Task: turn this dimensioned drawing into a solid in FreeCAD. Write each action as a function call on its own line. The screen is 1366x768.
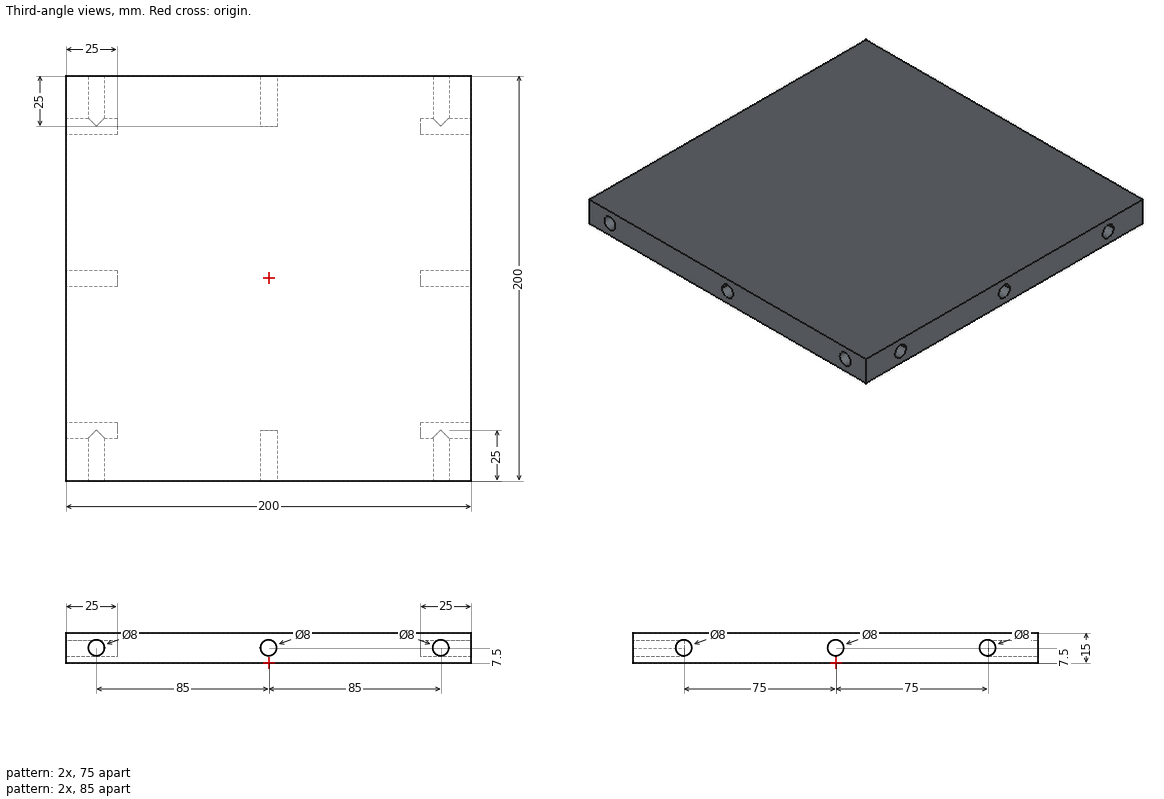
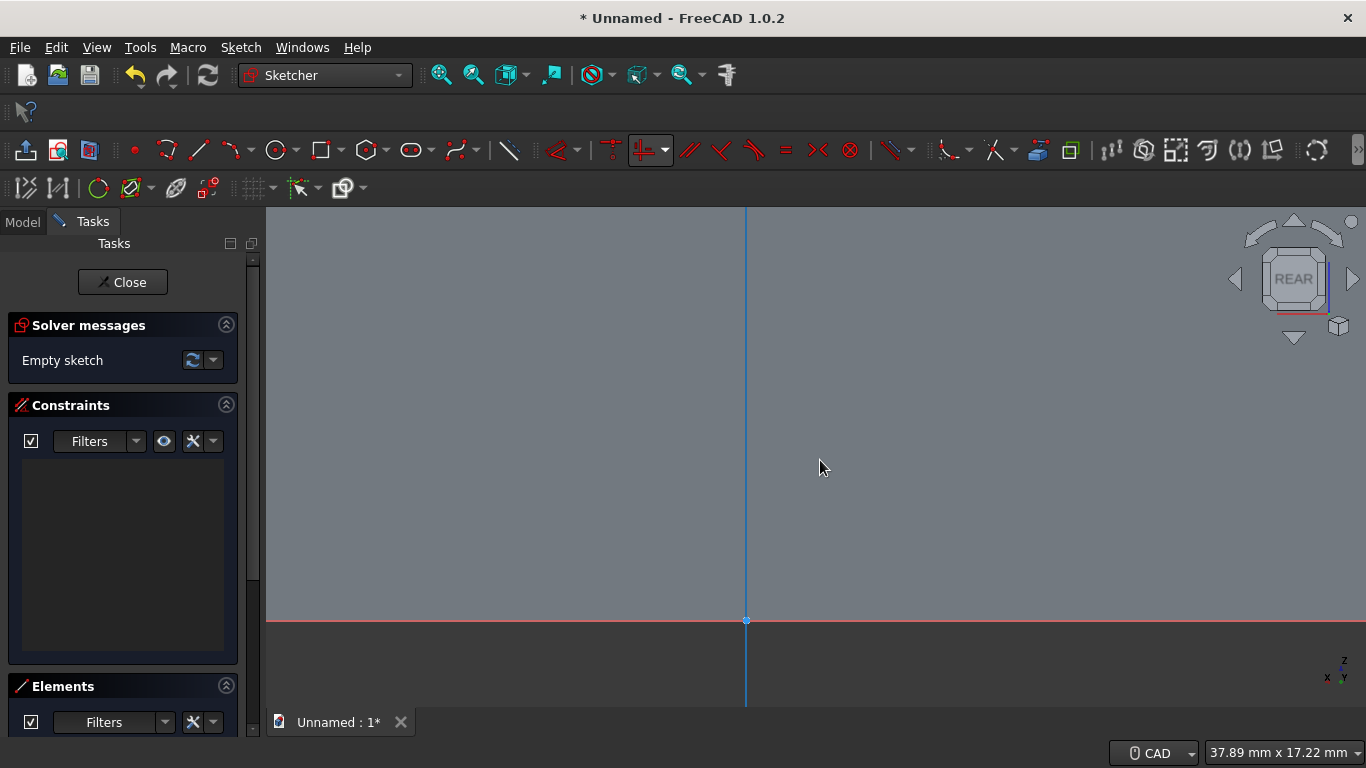
click(276, 150)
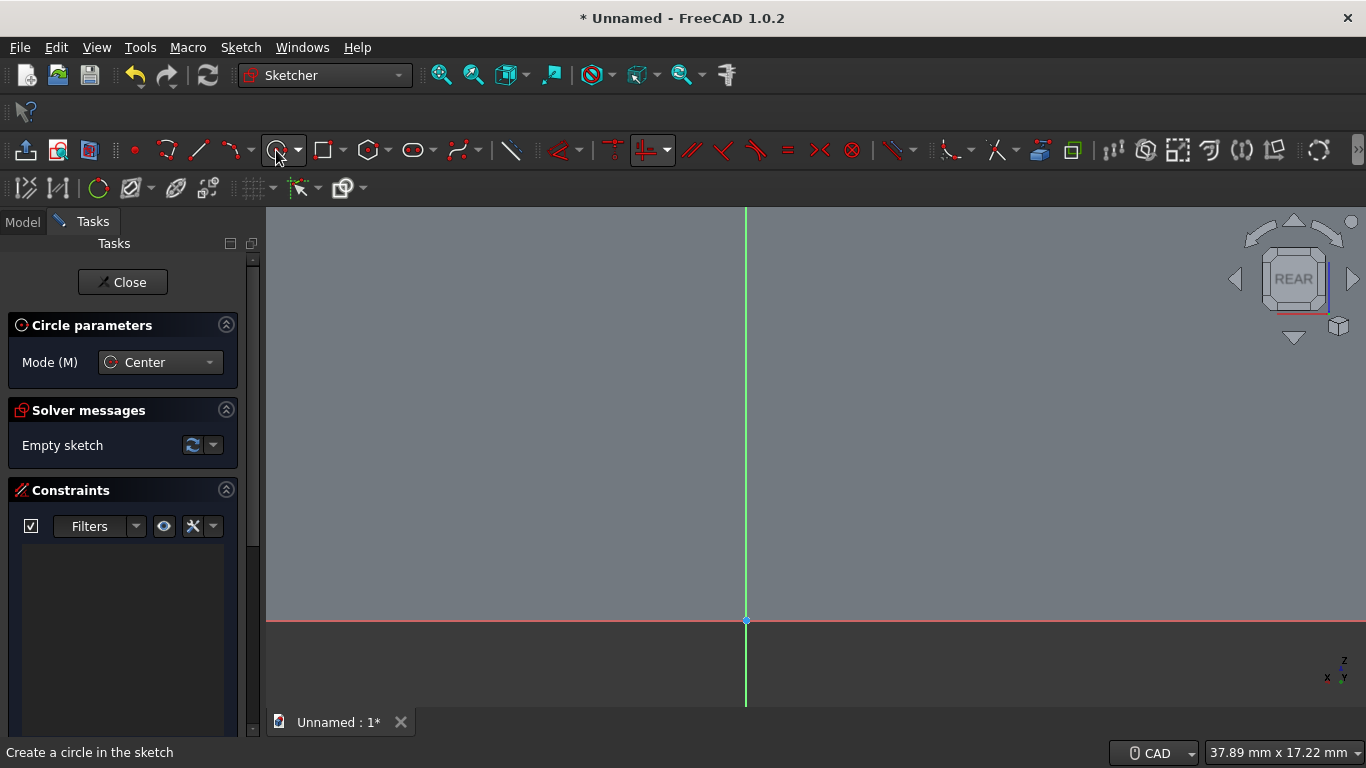
click(746, 403)
move(829, 321)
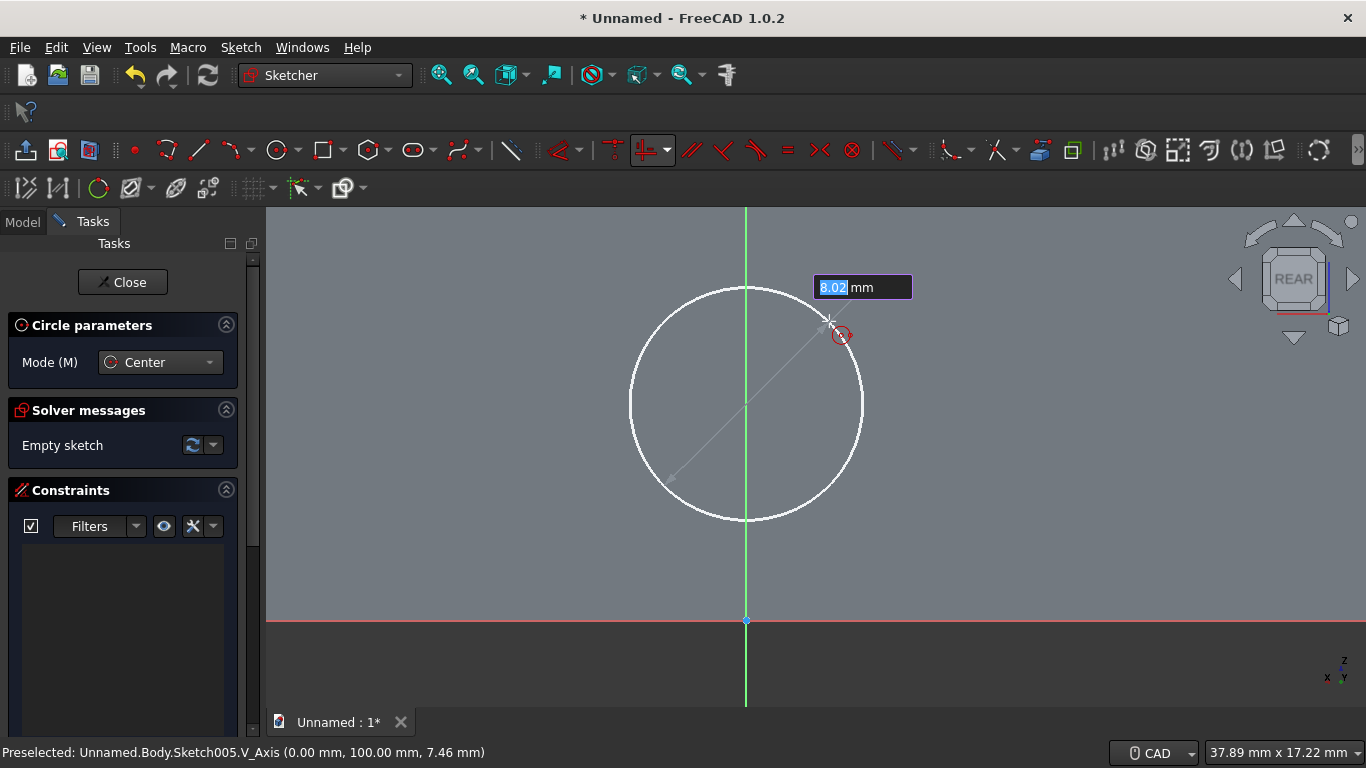
text(8)
key(Return)
key(Escape)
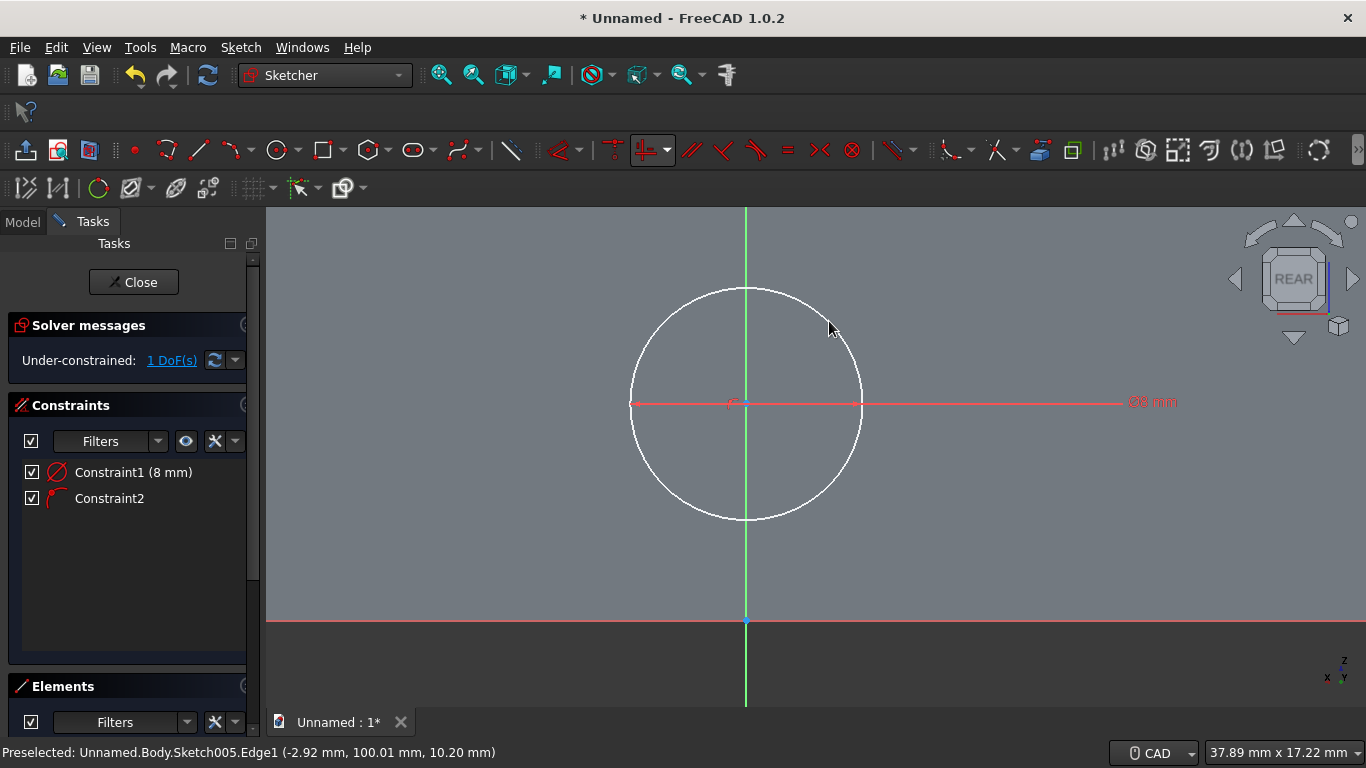
key(d)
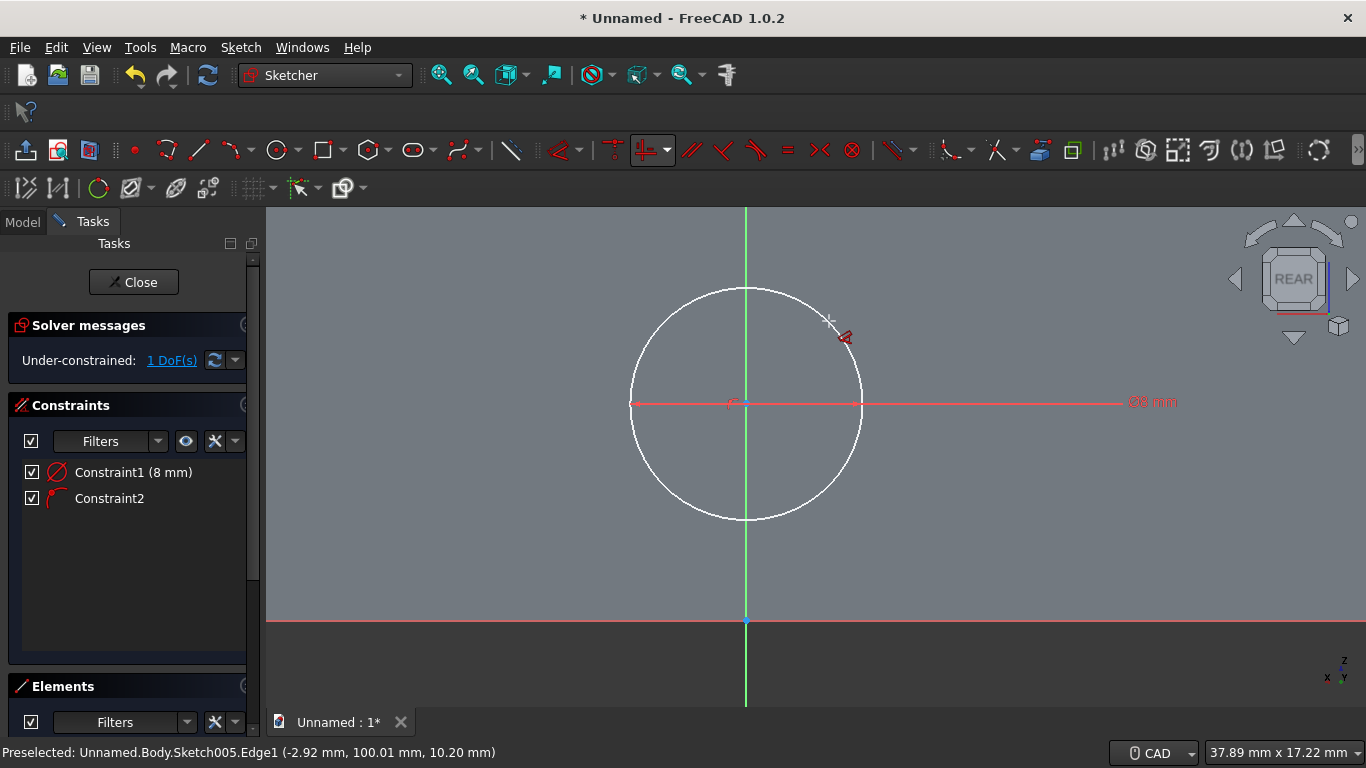
click(746, 404)
click(780, 462)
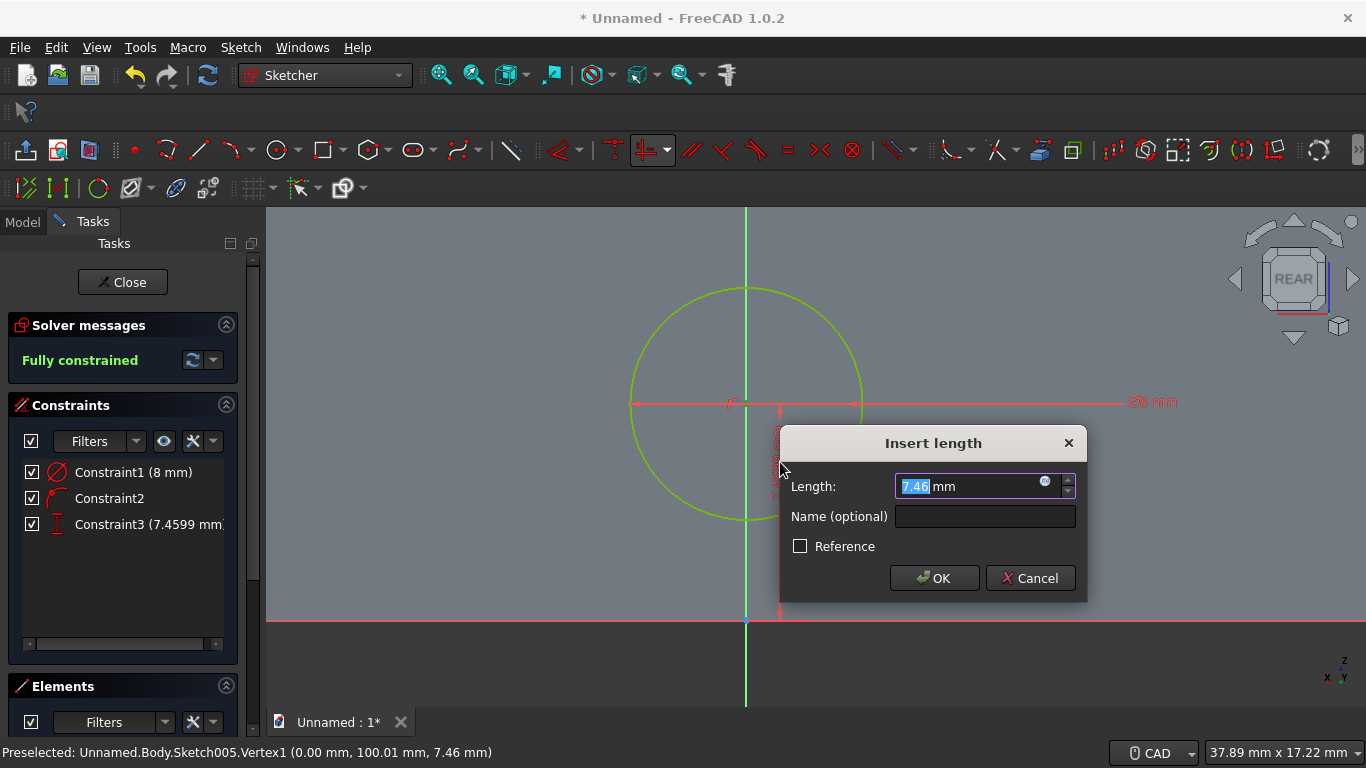
text(7.5)
key(Return)
key(Escape)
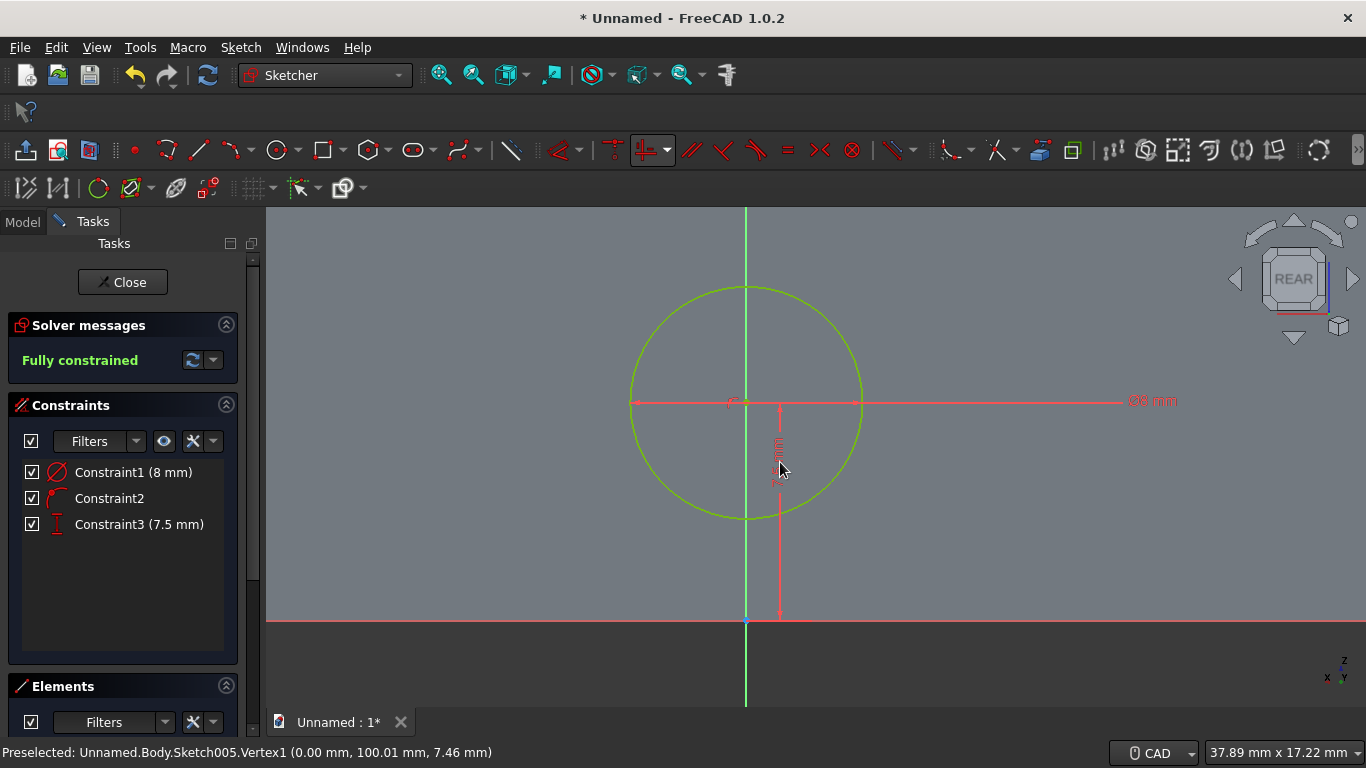
click(123, 282)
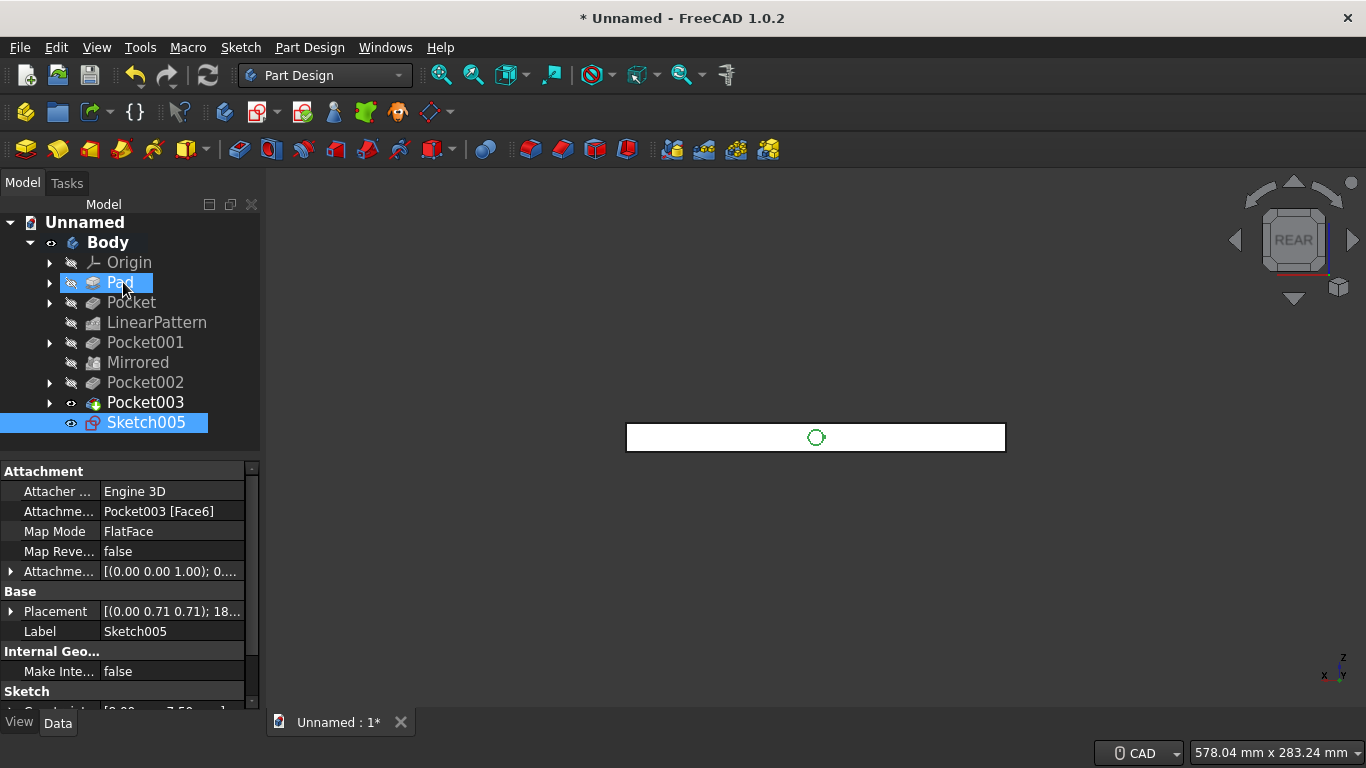
click(240, 150)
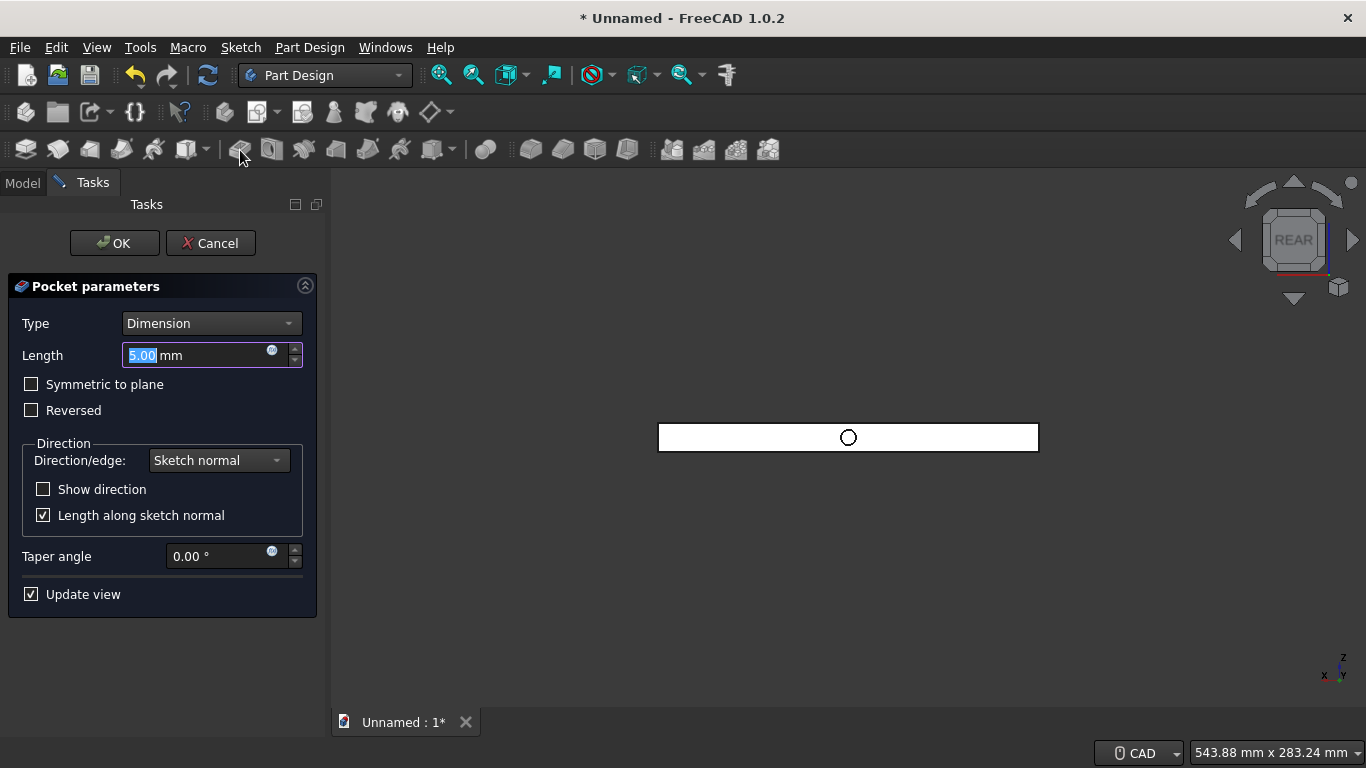
text(25)
key(Tab)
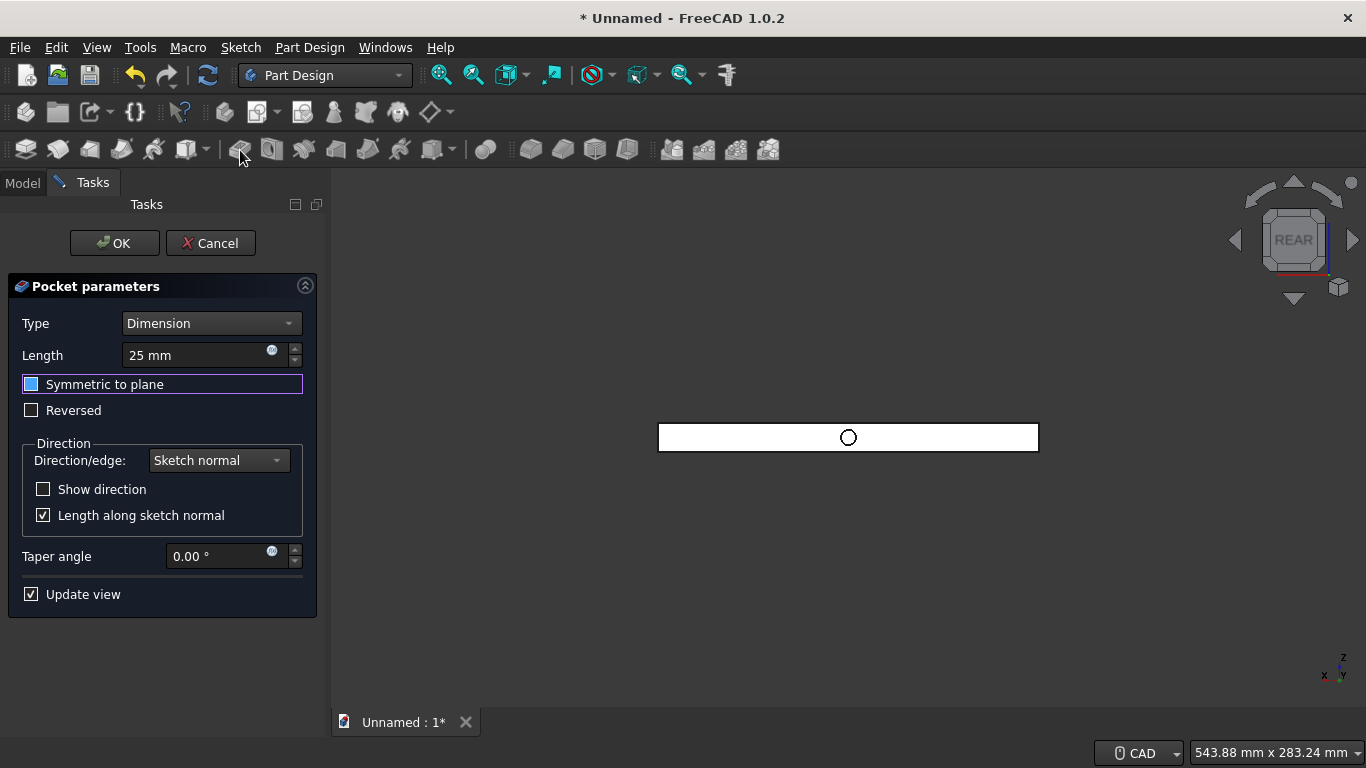
click(115, 243)